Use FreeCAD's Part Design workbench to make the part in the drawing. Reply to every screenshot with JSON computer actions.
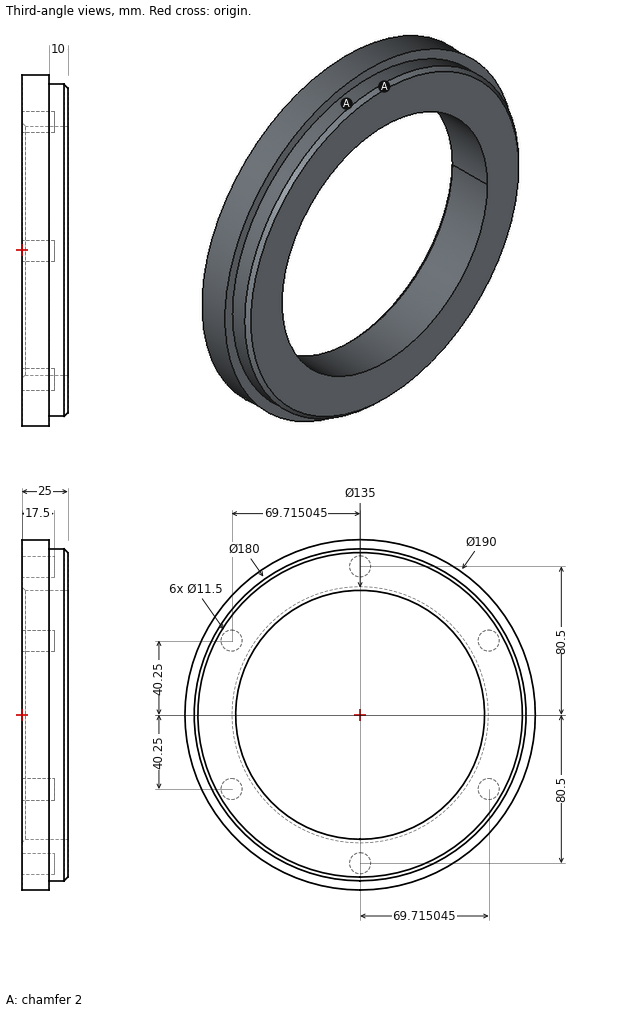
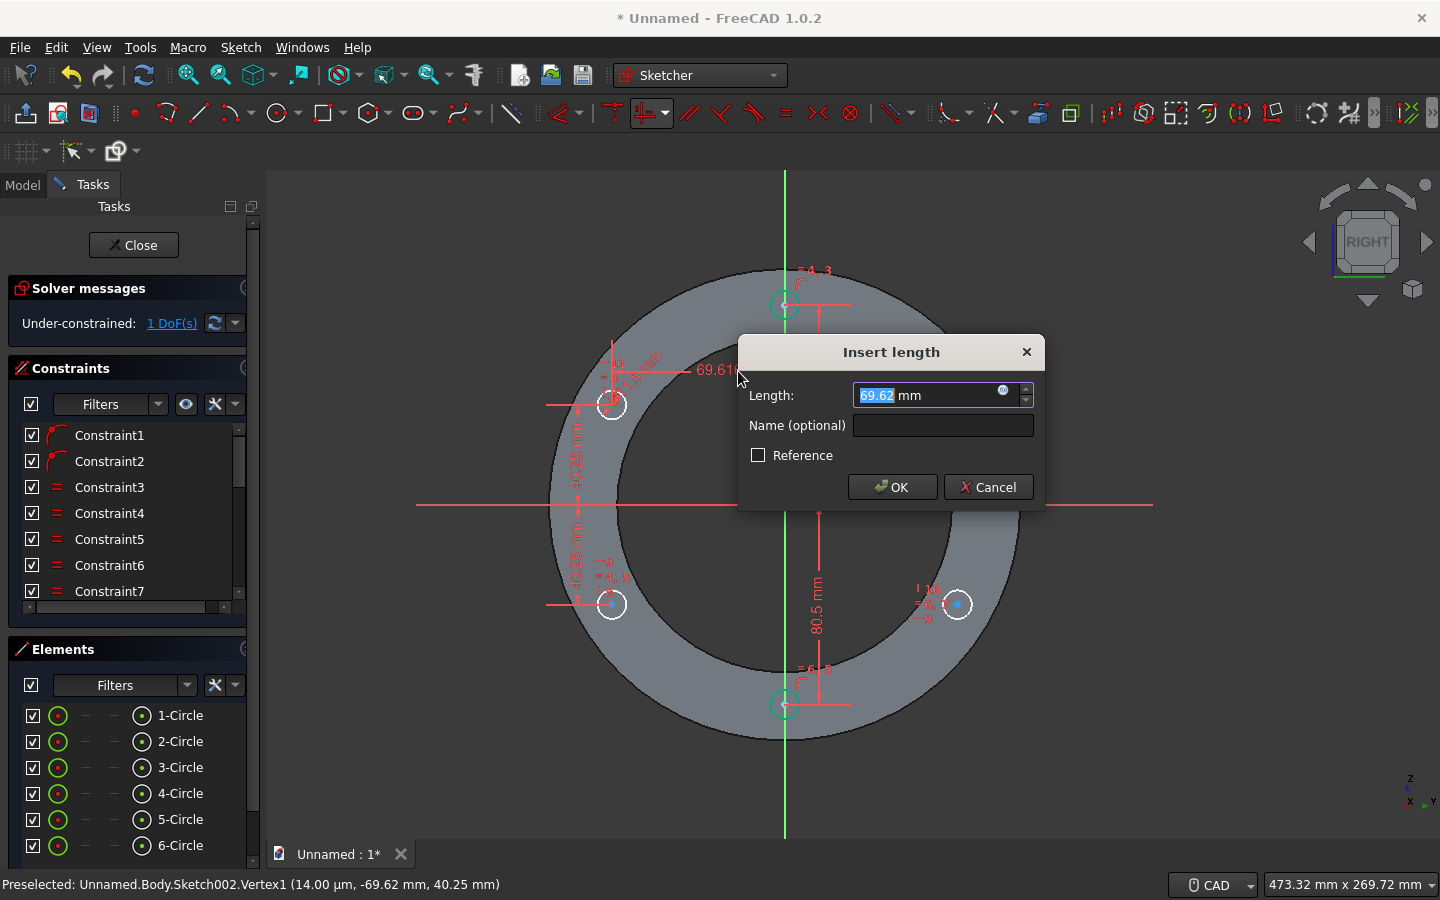
{"action": "type", "text": "69.715045"}
{"action": "key", "text": "Return"}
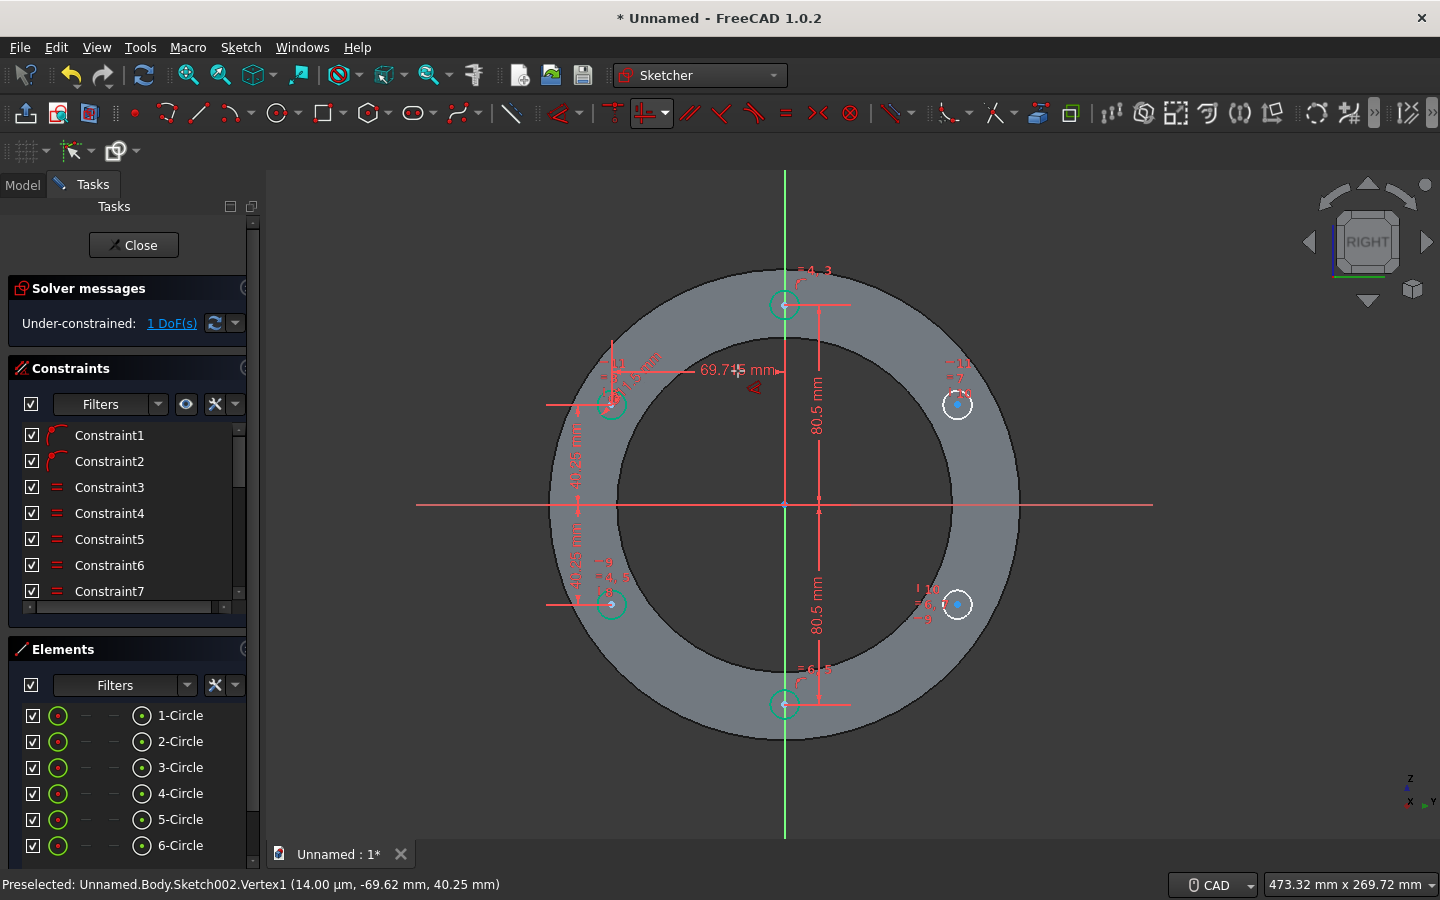
{"action": "left_click", "coordinate": [958, 605]}
{"action": "left_click", "coordinate": [871, 639]}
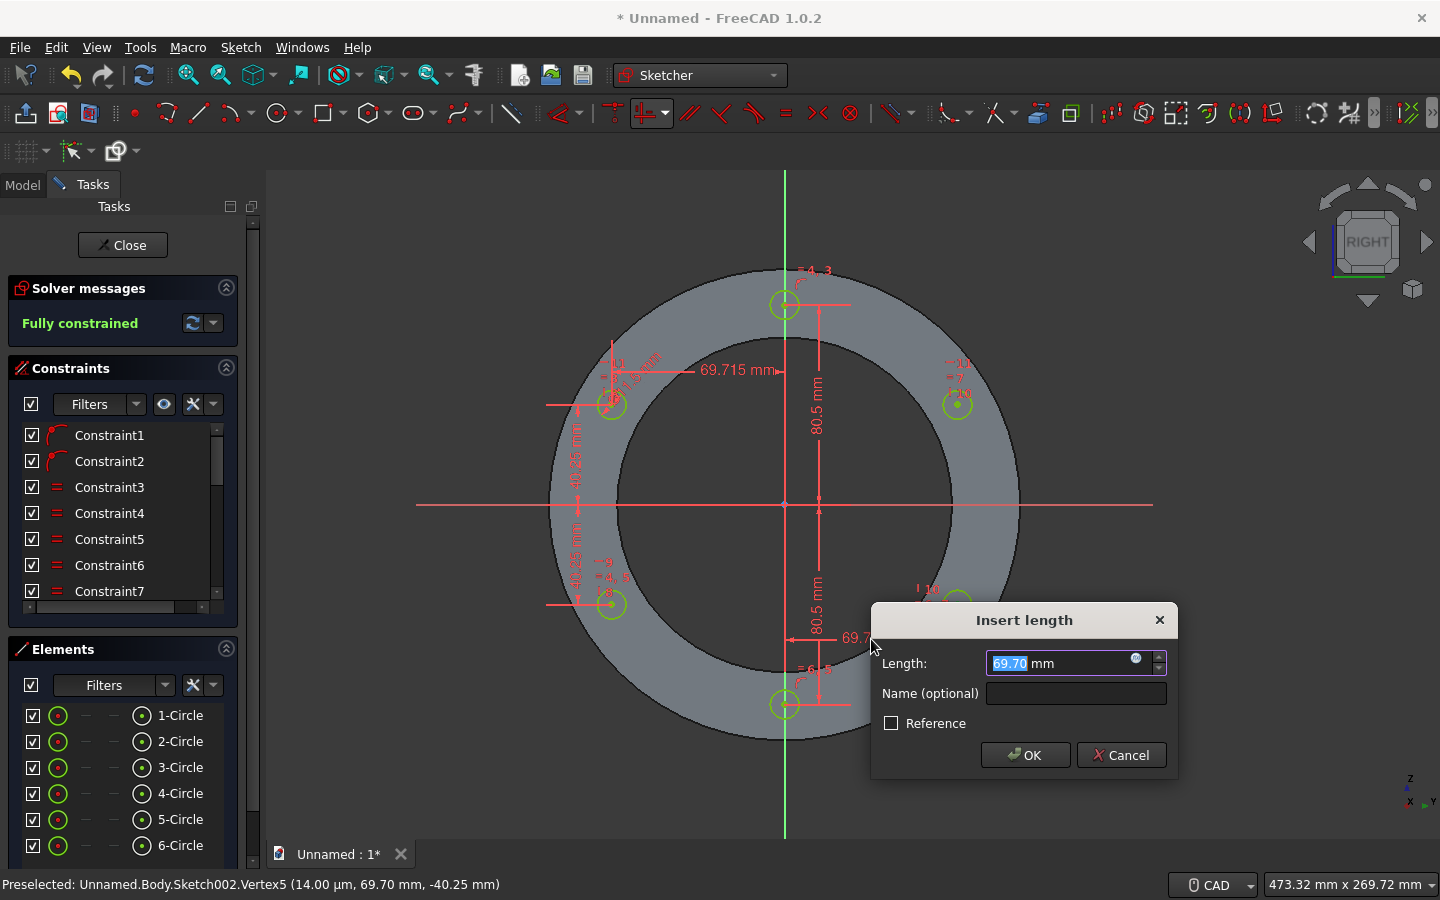
{"action": "type", "text": "69.715045"}
{"action": "key", "text": "Return"}
{"action": "key", "text": "Escape"}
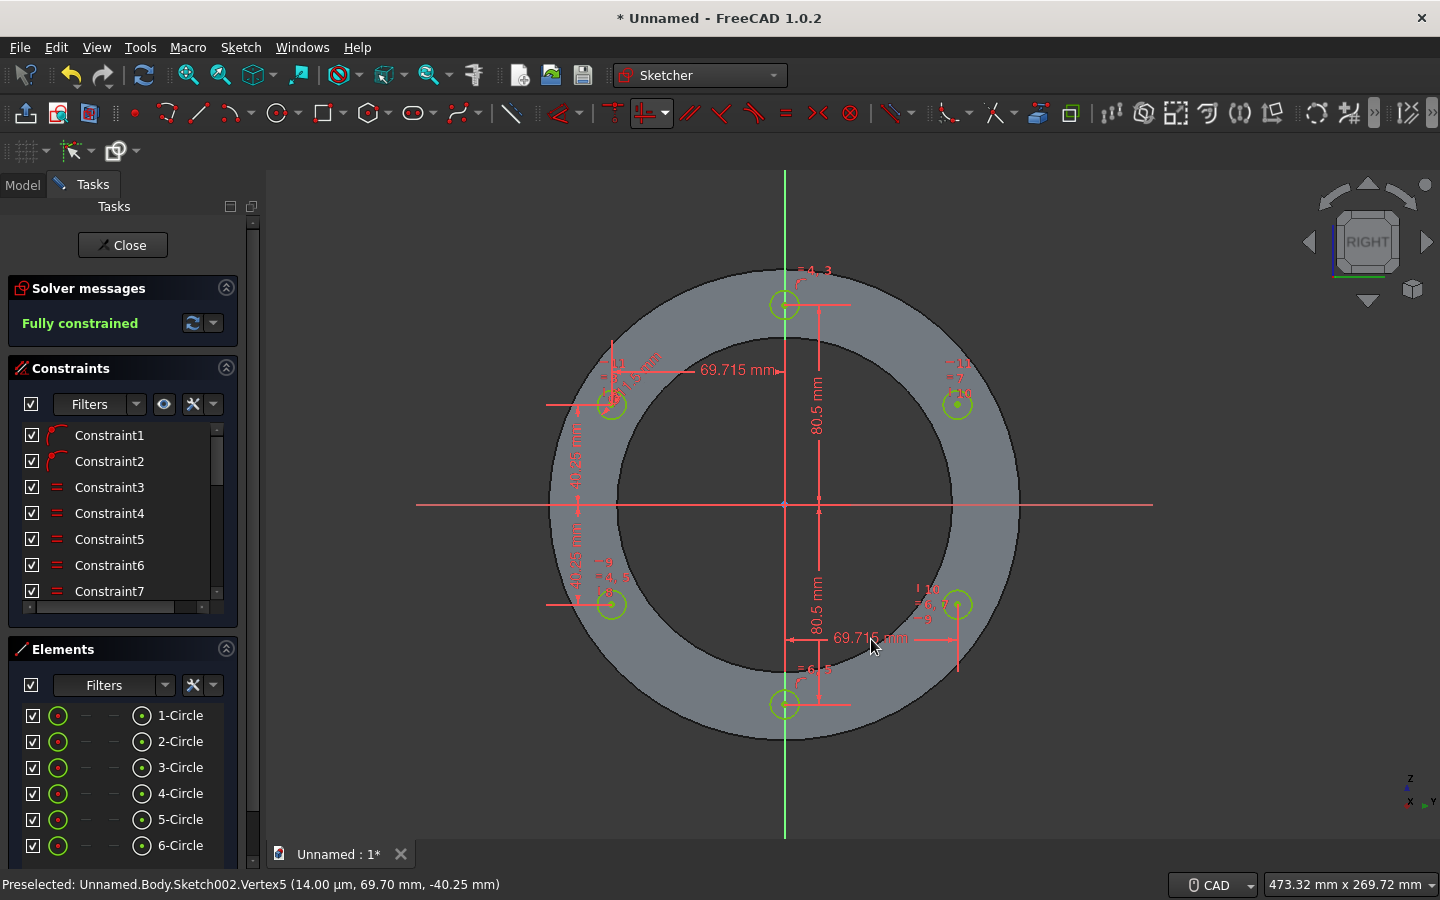
{"action": "left_click", "coordinate": [123, 245]}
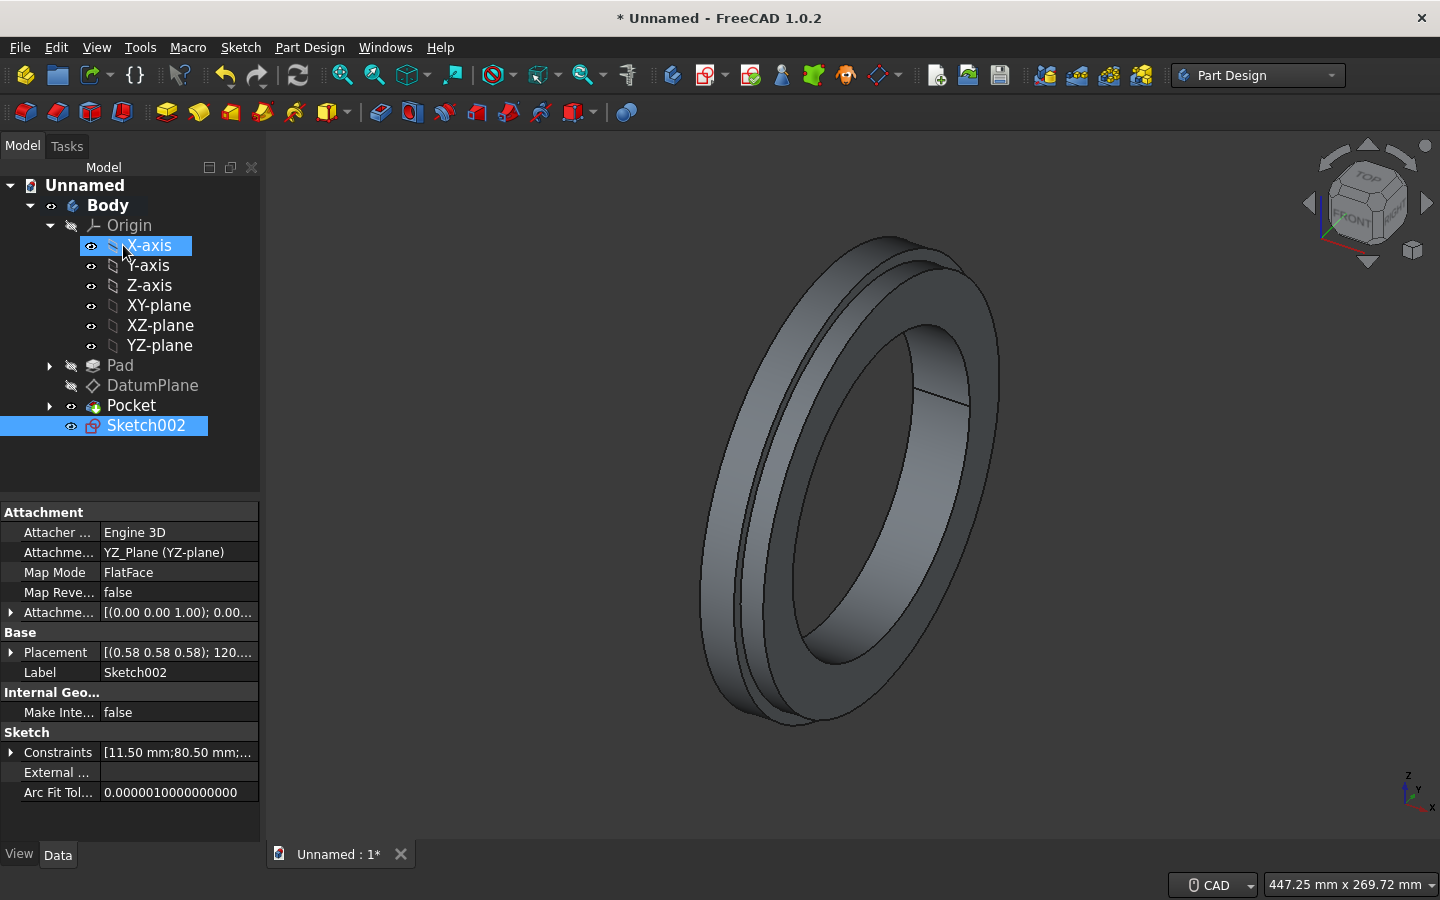
{"action": "left_click", "coordinate": [382, 112]}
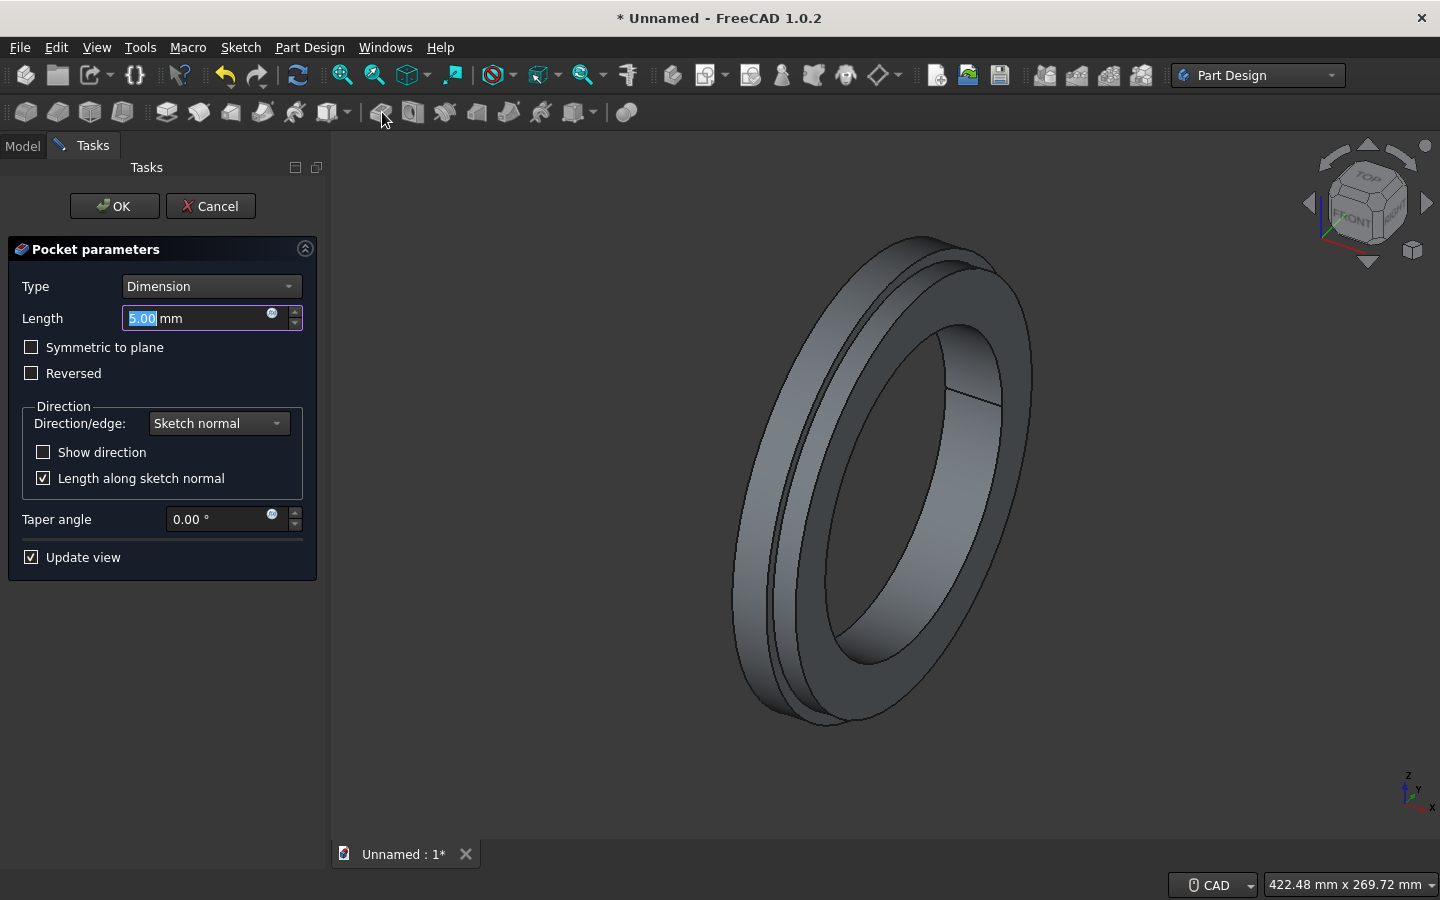
{"action": "type", "text": "17.5"}
{"action": "key", "text": "Tab"}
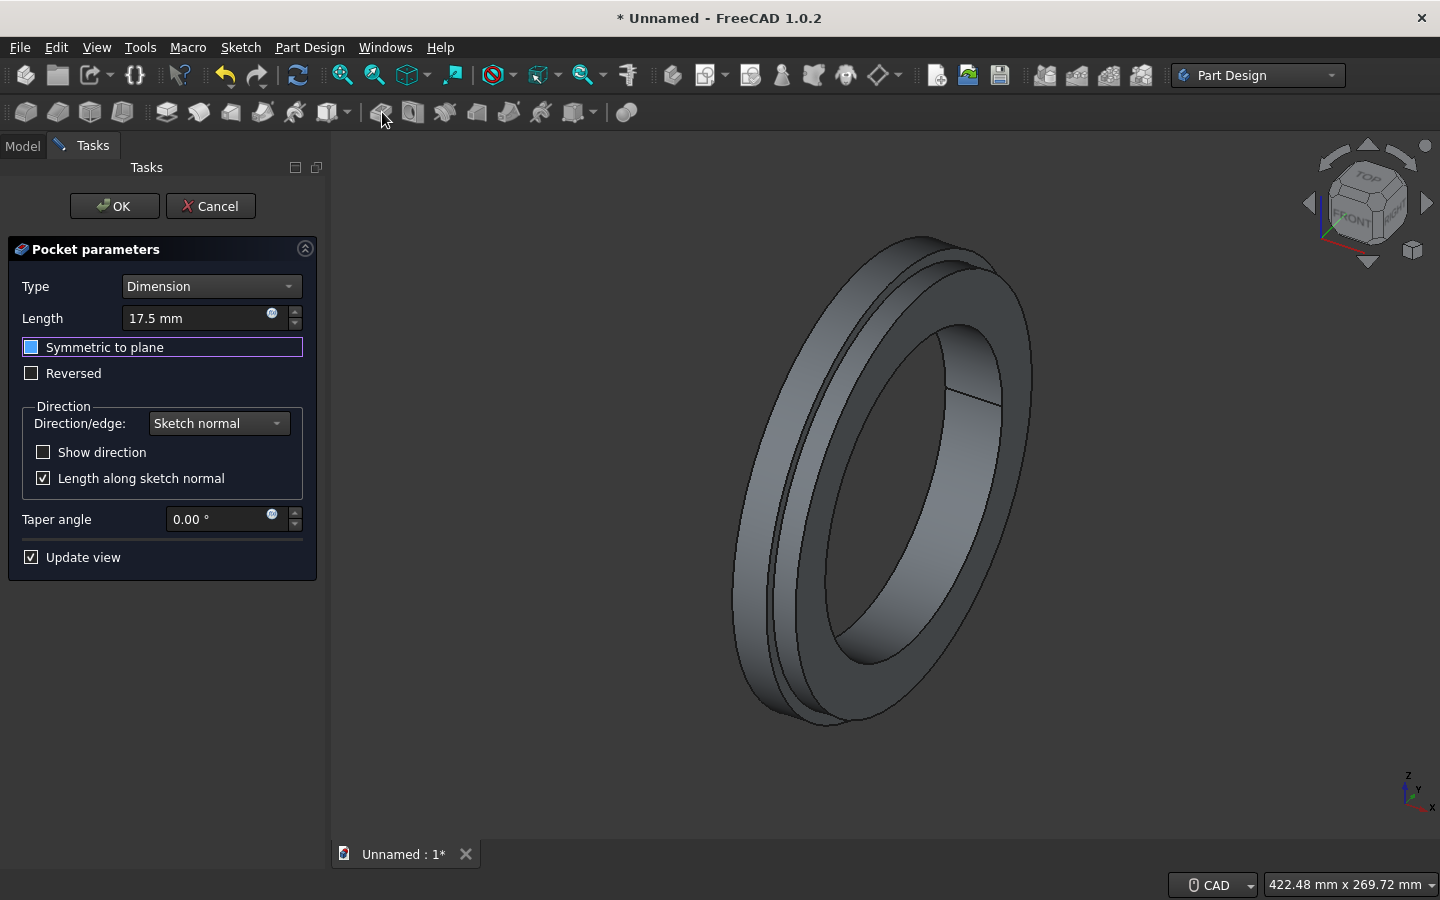
{"action": "left_click", "coordinate": [30, 373]}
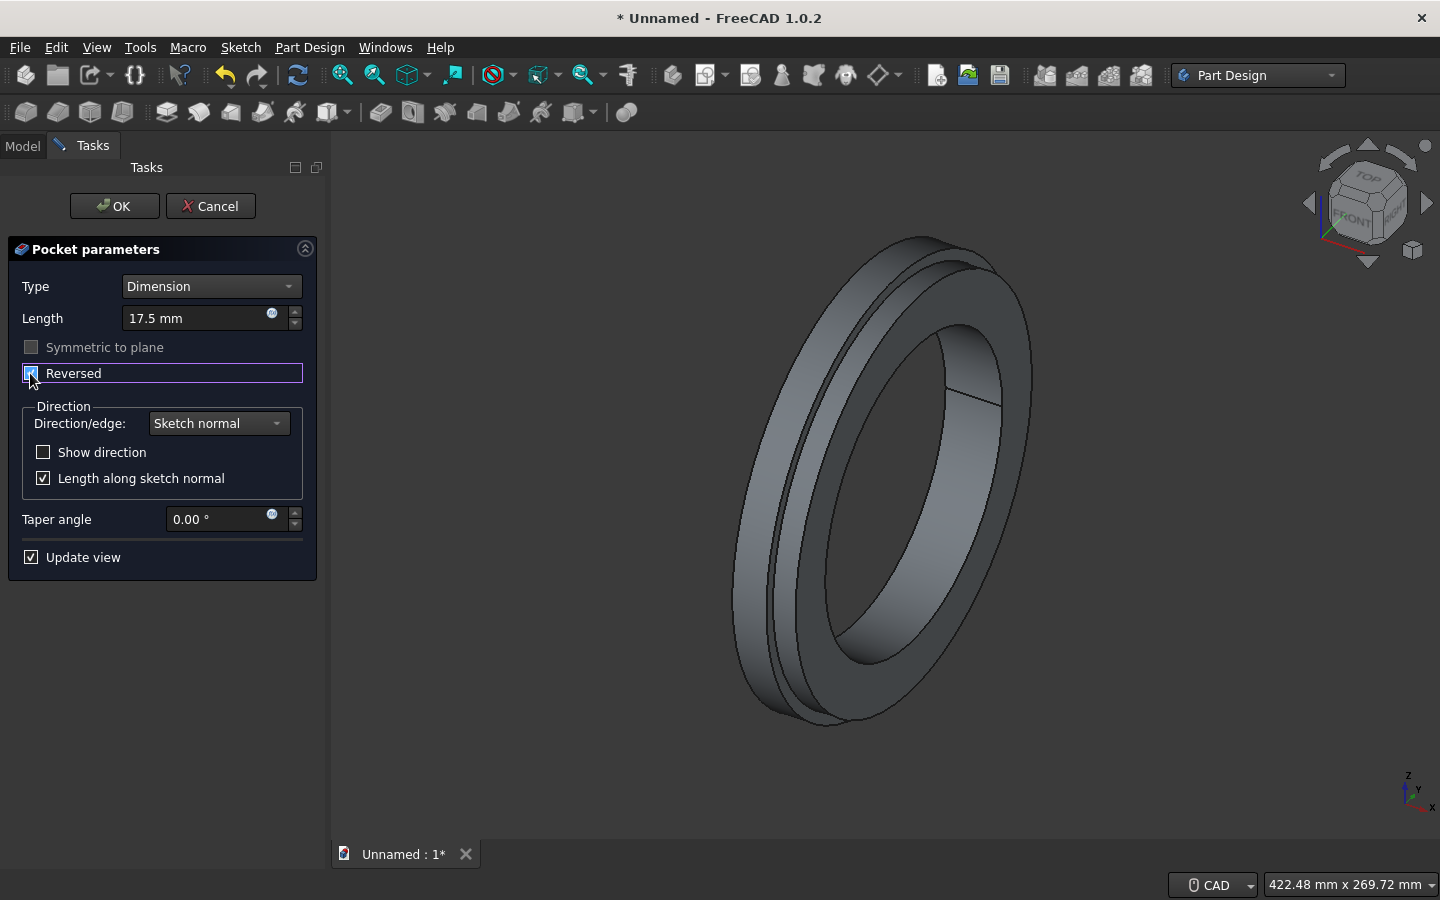
{"action": "left_click", "coordinate": [115, 206]}